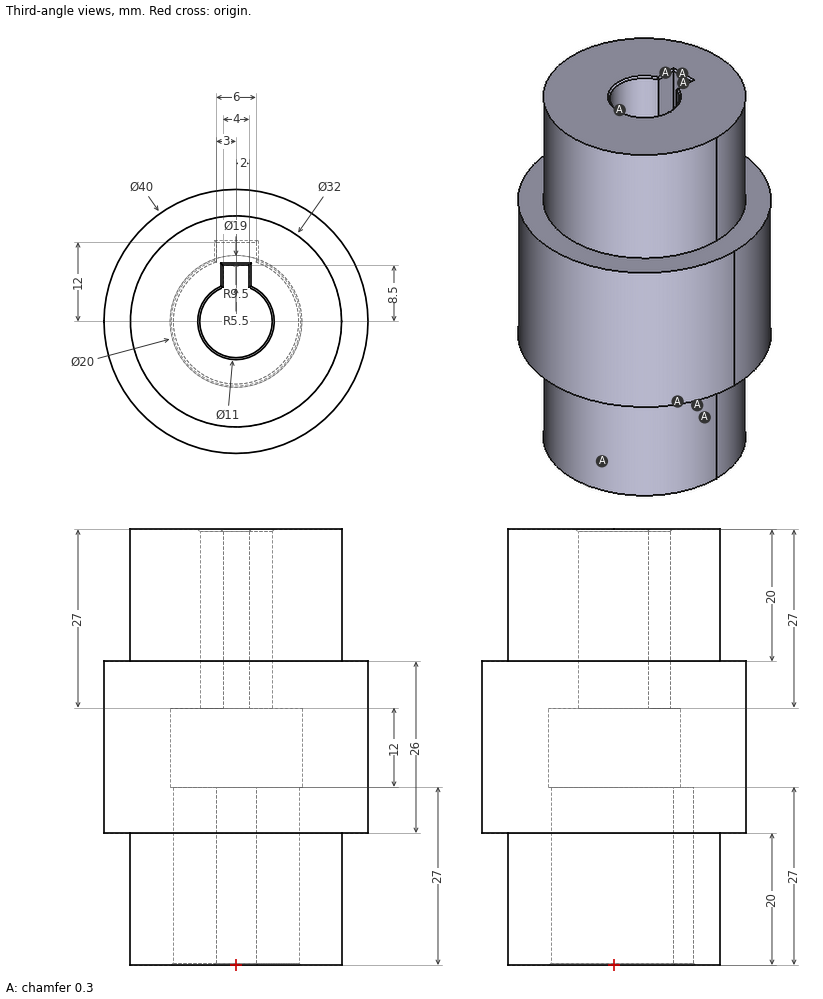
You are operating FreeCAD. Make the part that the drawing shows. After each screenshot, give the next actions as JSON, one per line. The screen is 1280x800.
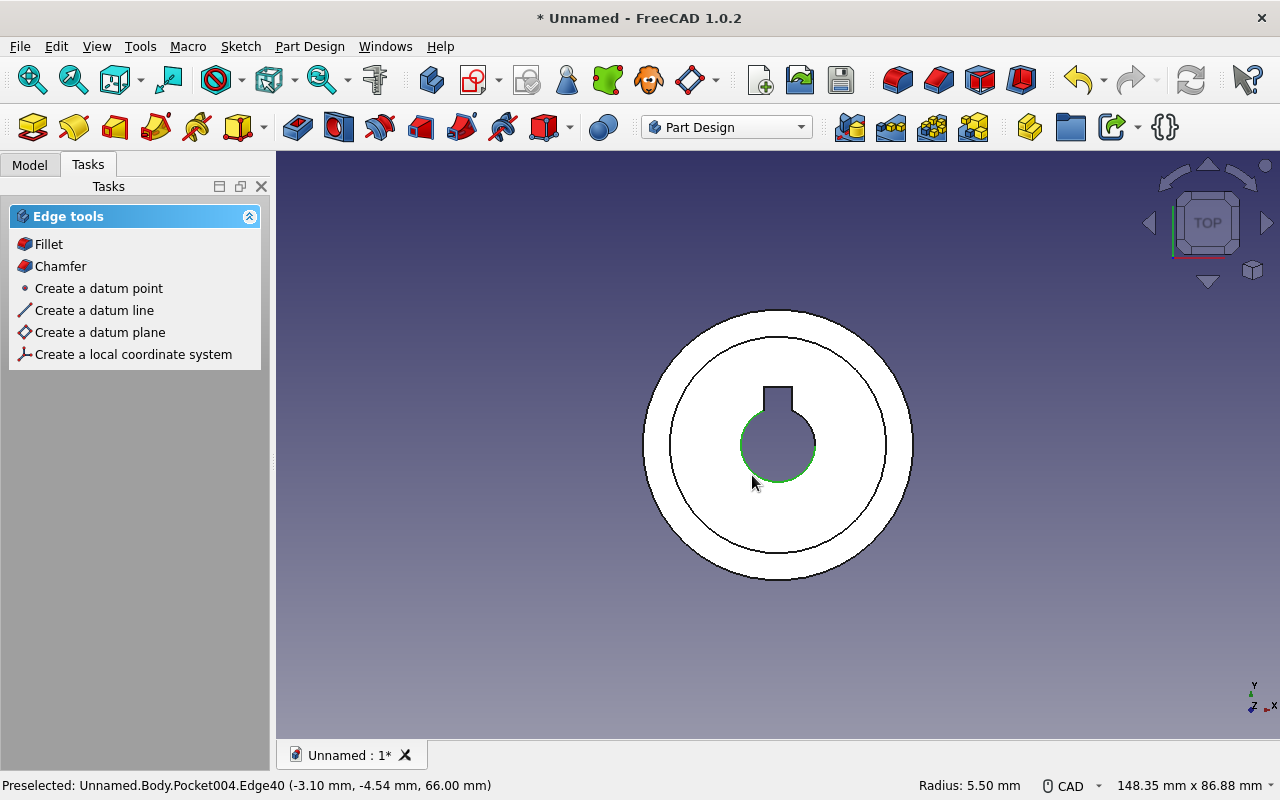
{"action": "left_click", "coordinate": [778, 386], "text": "ctrl"}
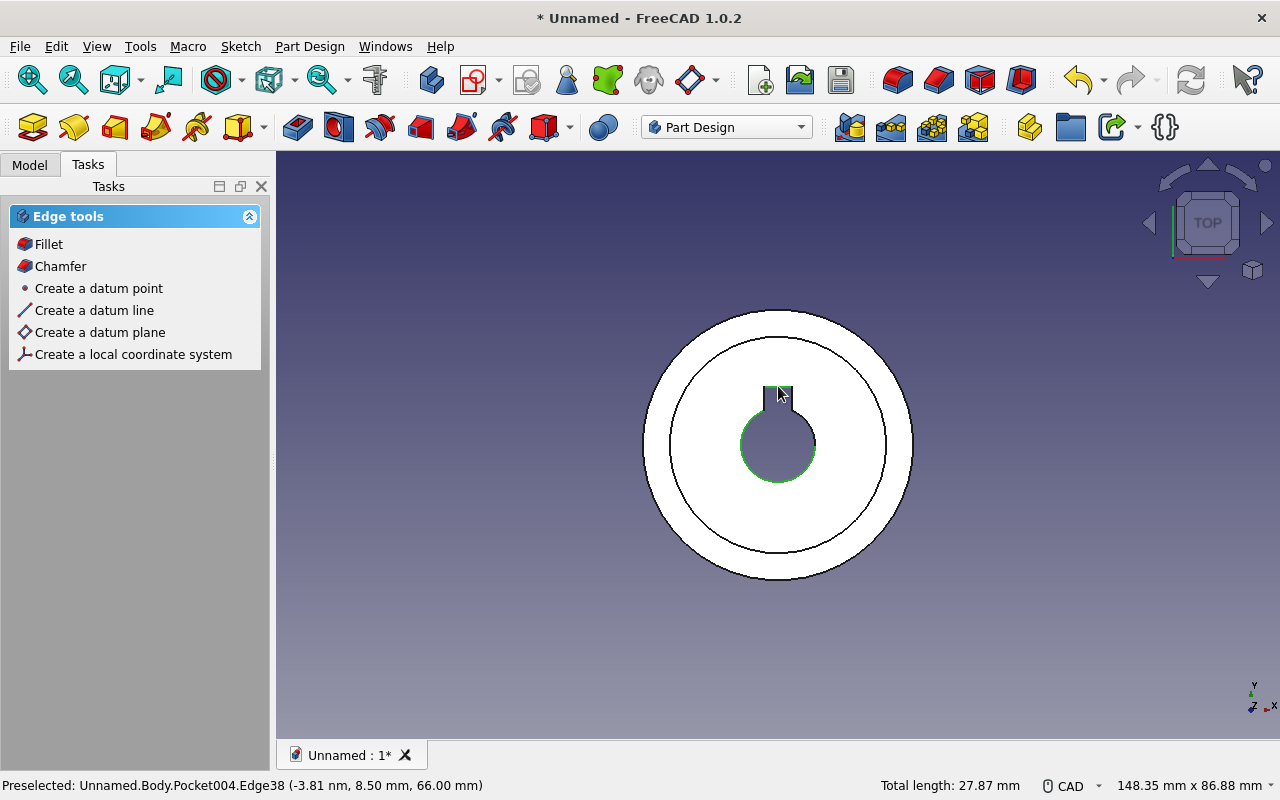
{"action": "left_click", "coordinate": [764, 398], "text": "ctrl"}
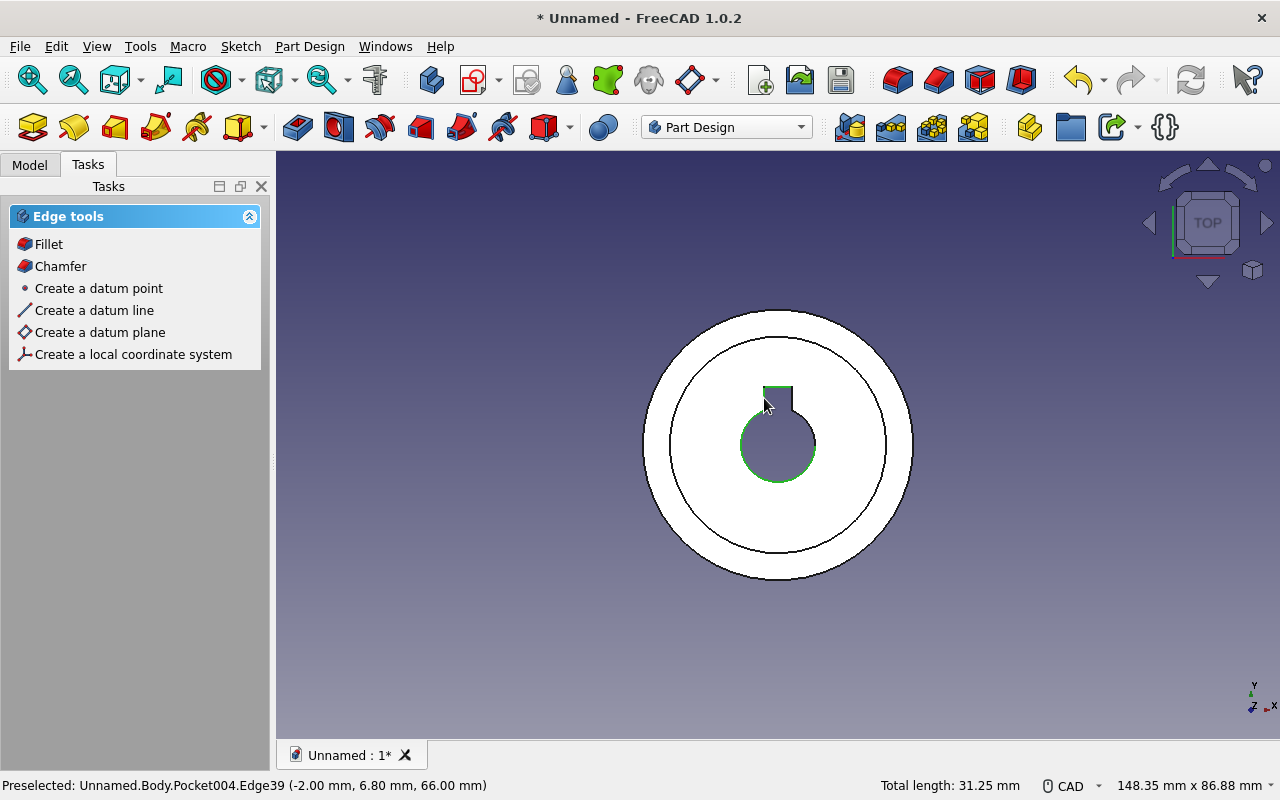
{"action": "left_click", "coordinate": [792, 398], "text": "ctrl"}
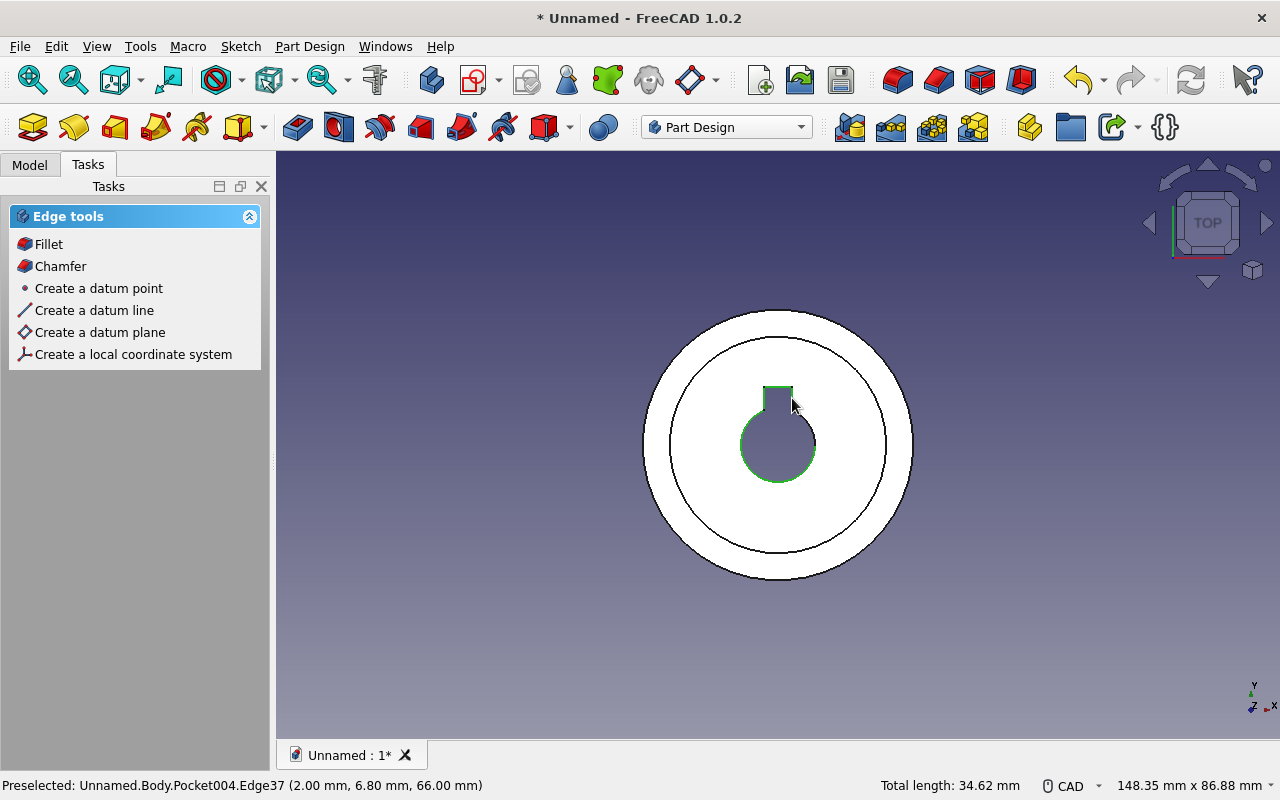
{"action": "key", "text": "0"}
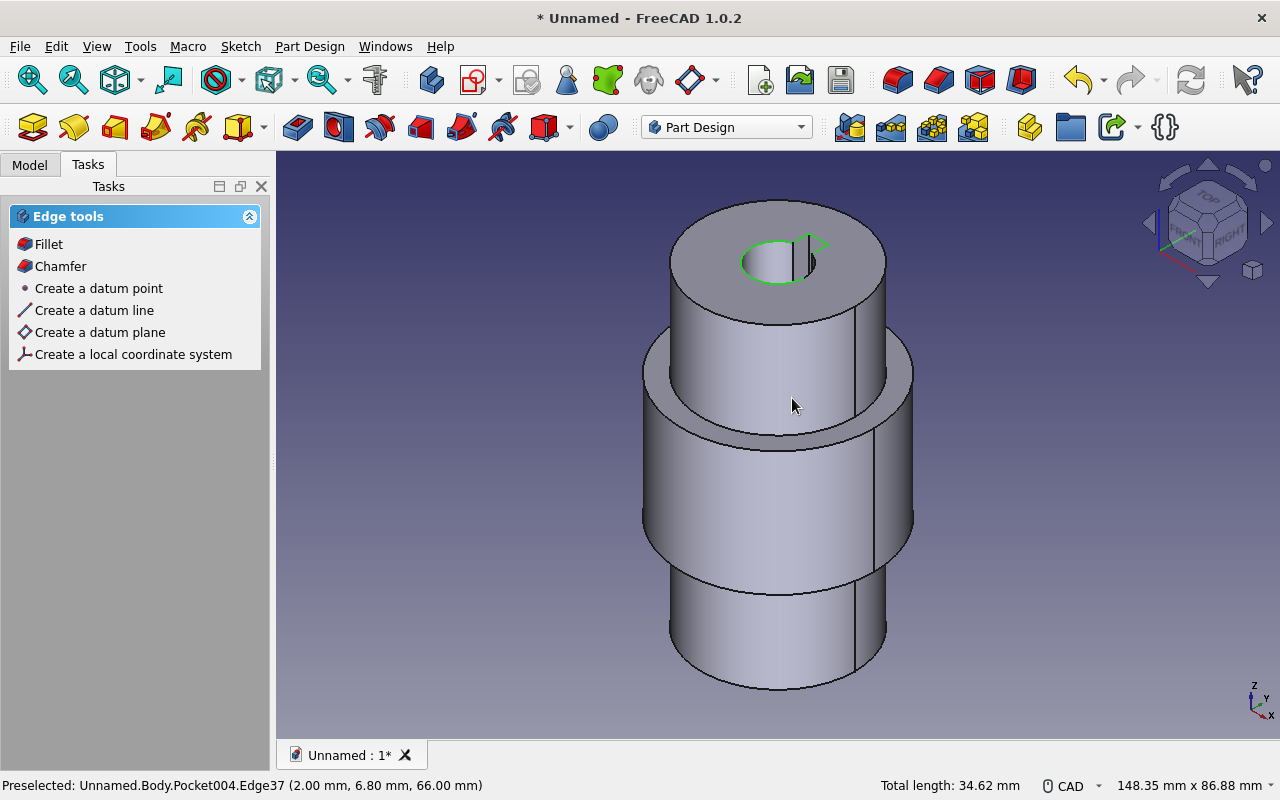
{"action": "key", "text": "2"}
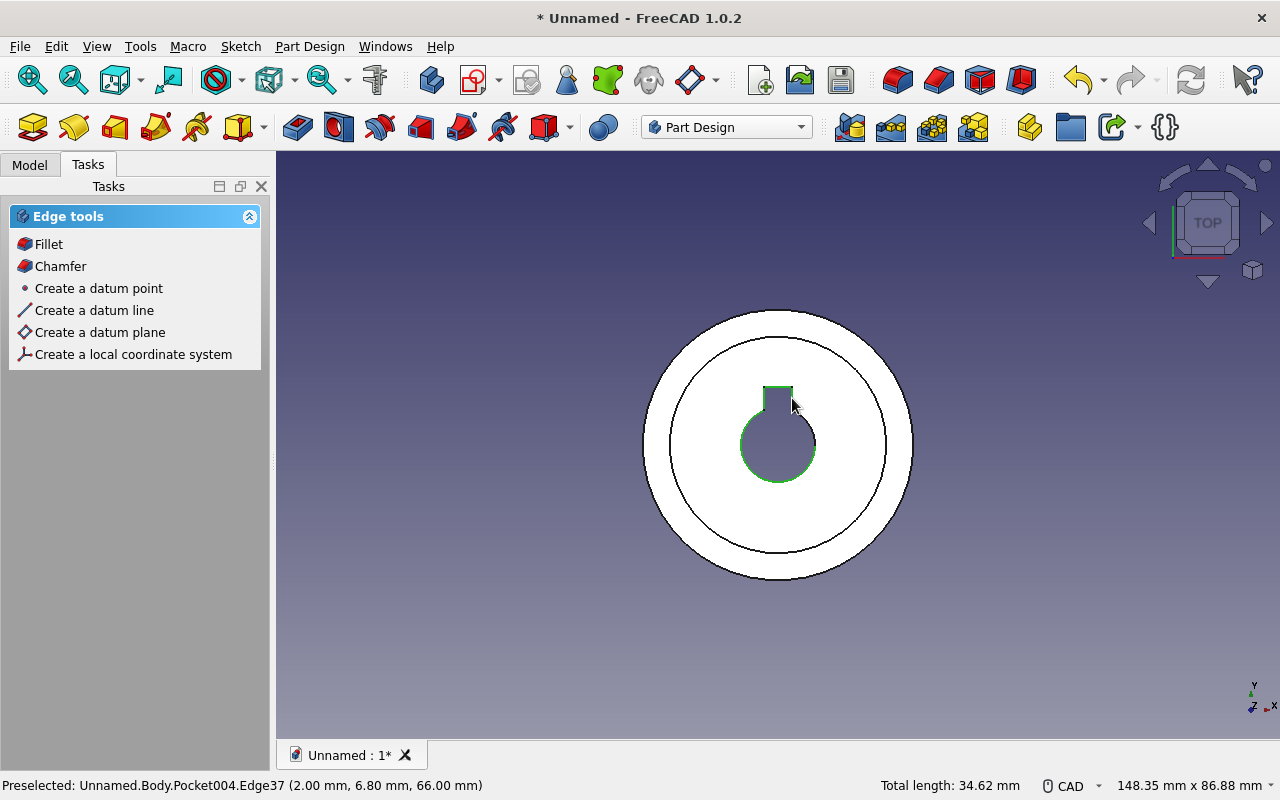
{"action": "key", "text": "1"}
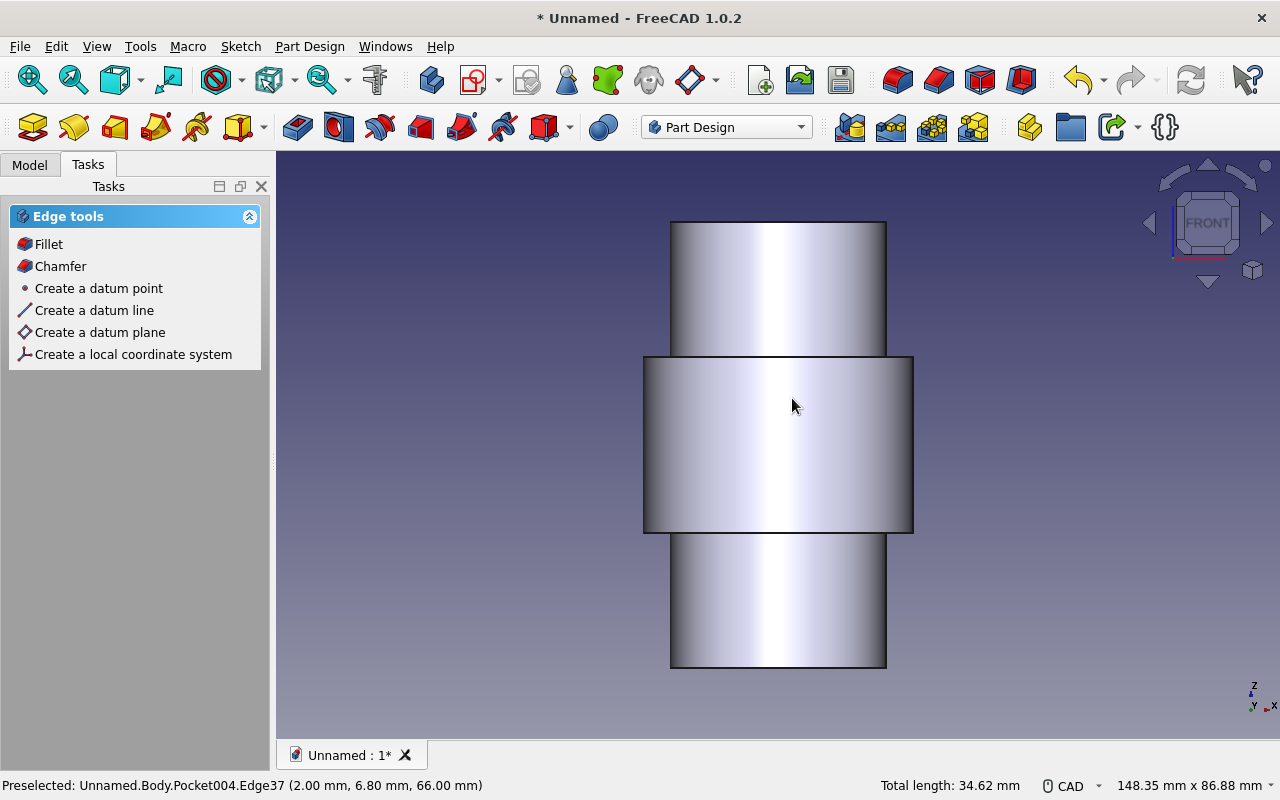
{"action": "key", "text": "3"}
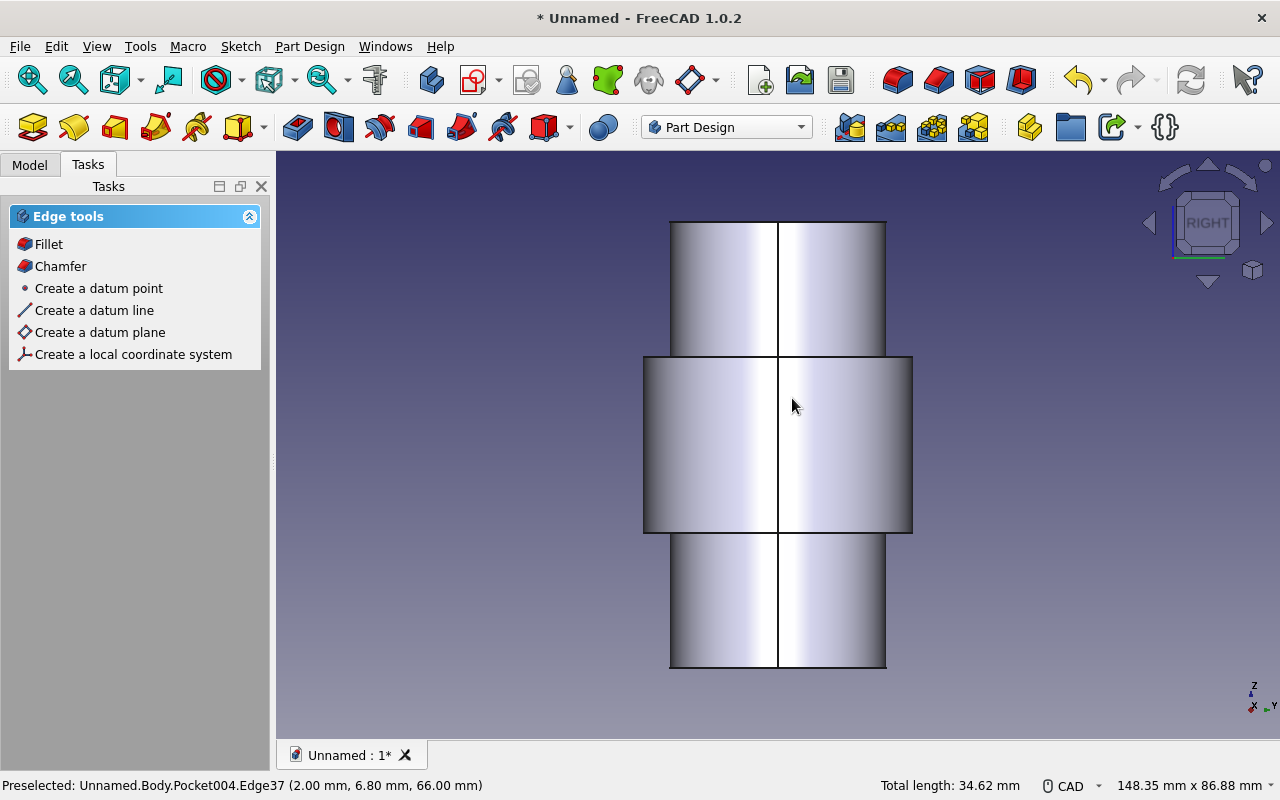
{"action": "key", "text": "5"}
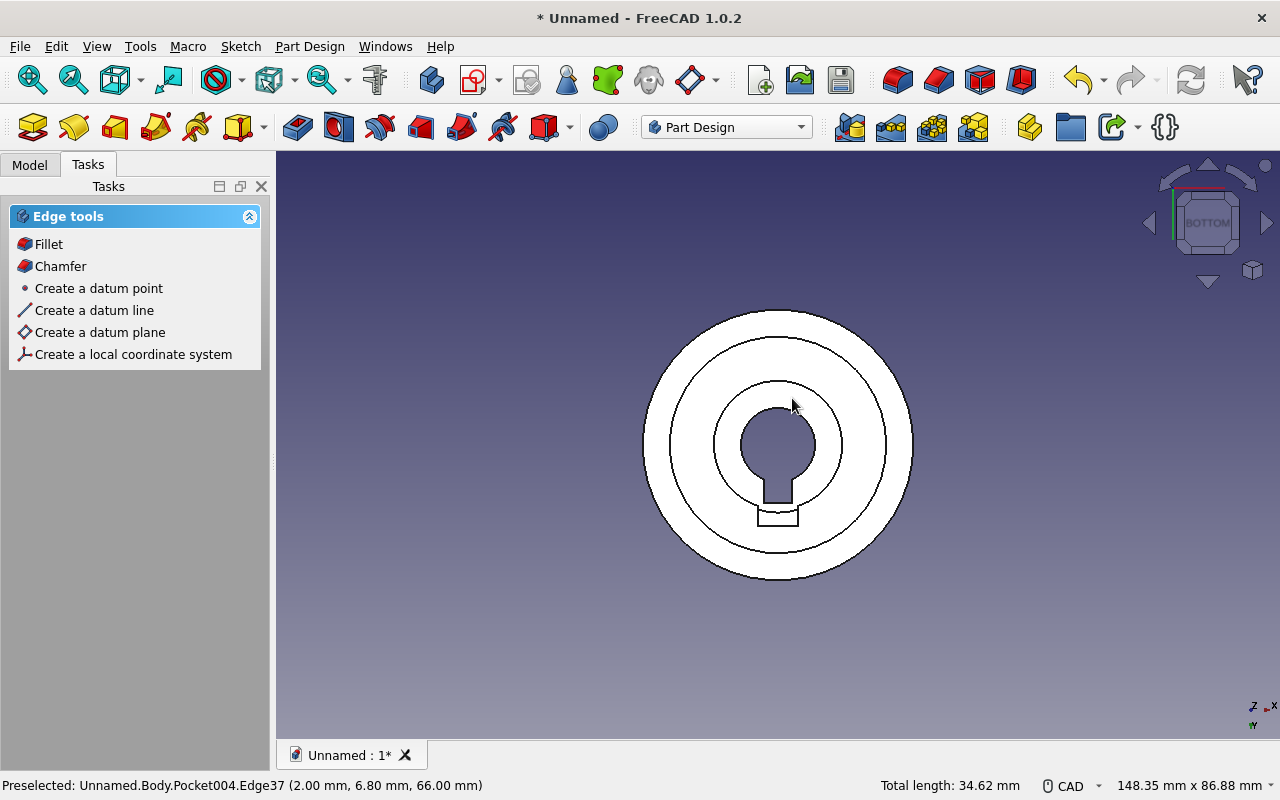
{"action": "left_click", "coordinate": [740, 392], "text": "ctrl"}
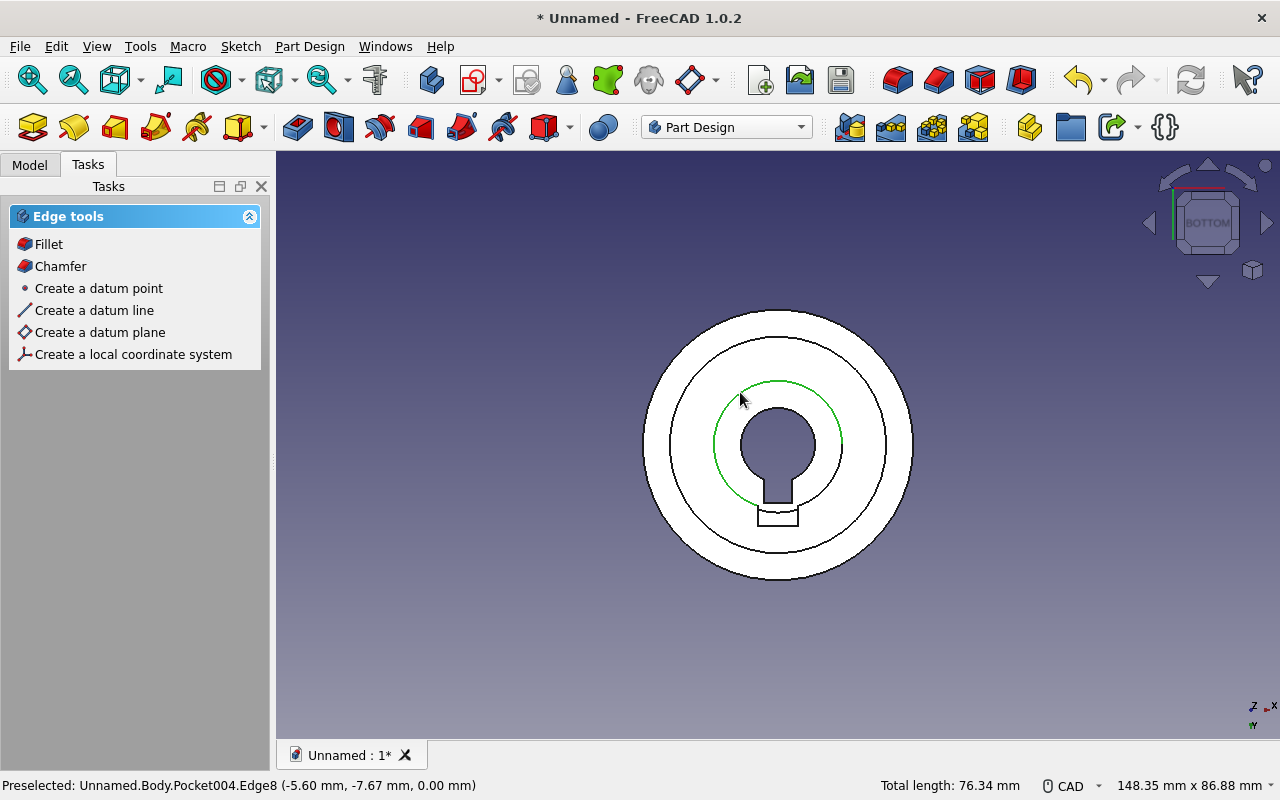
{"action": "left_click", "coordinate": [778, 525], "text": "ctrl"}